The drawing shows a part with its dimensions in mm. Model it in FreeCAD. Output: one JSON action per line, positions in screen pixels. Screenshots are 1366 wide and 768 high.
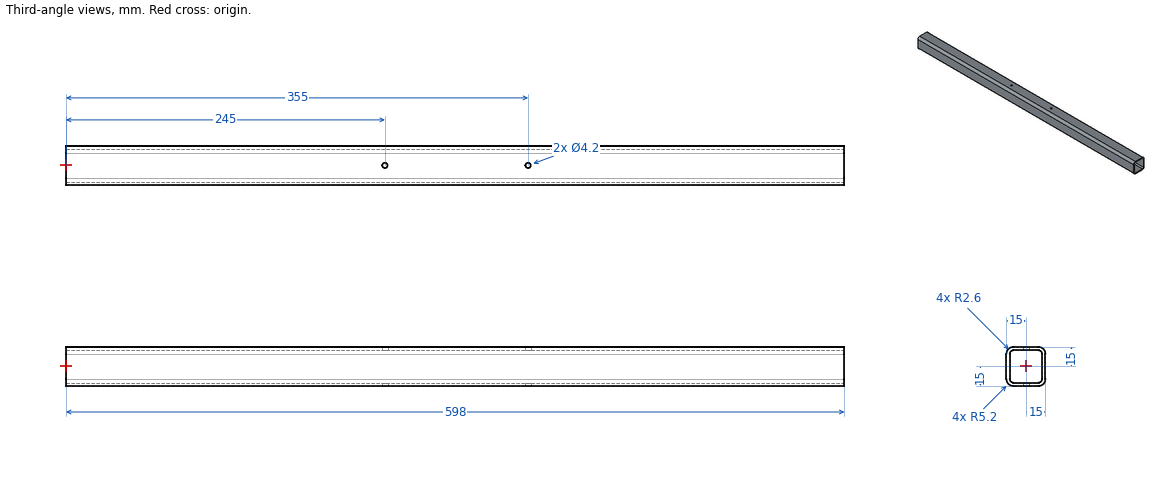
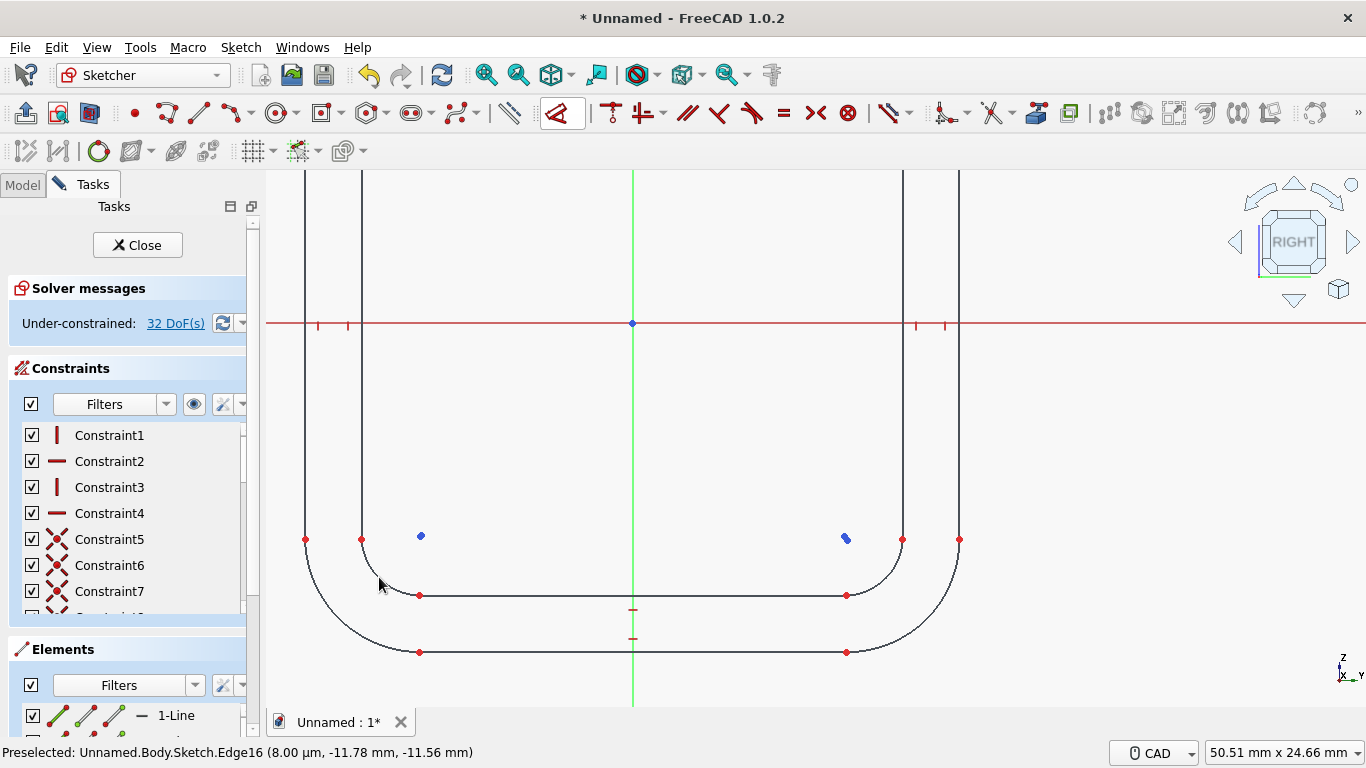
{"action": "left_click", "coordinate": [305, 239]}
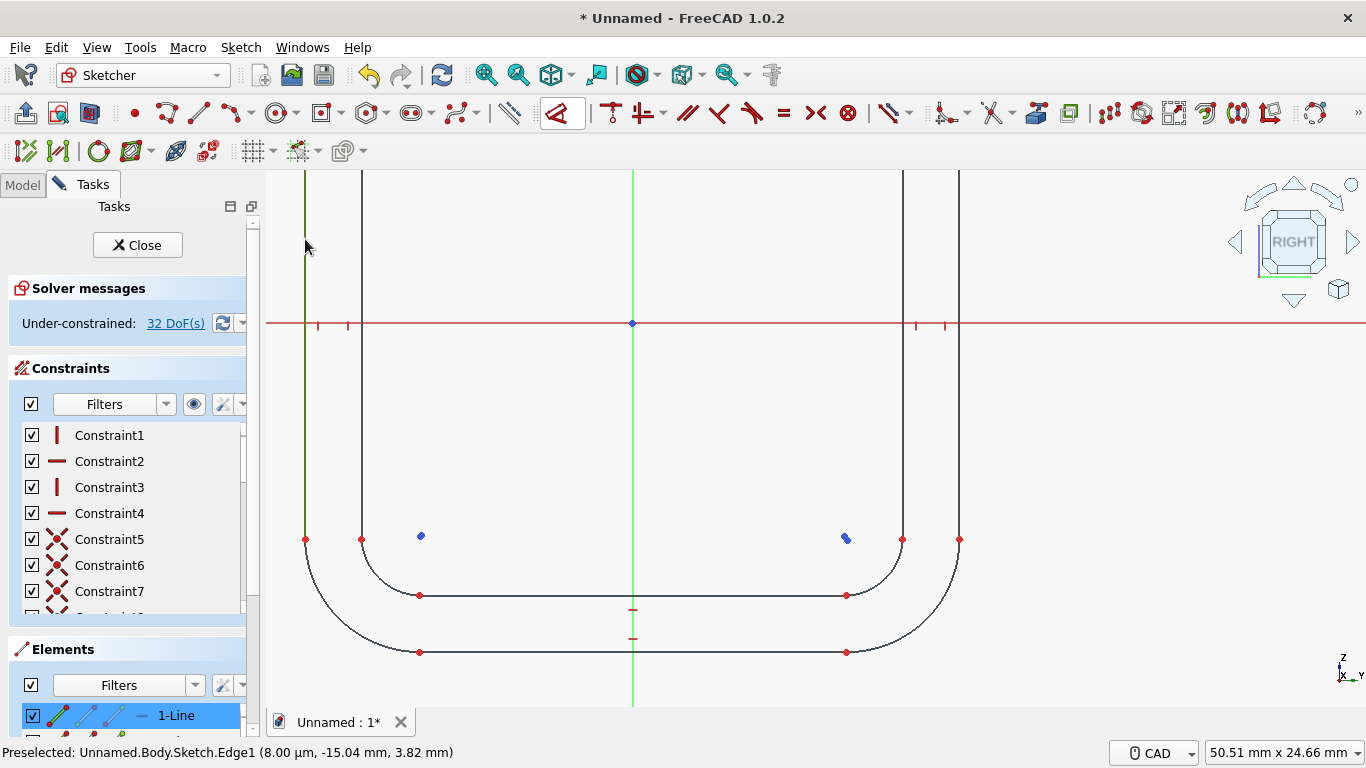
{"action": "left_click", "coordinate": [318, 590]}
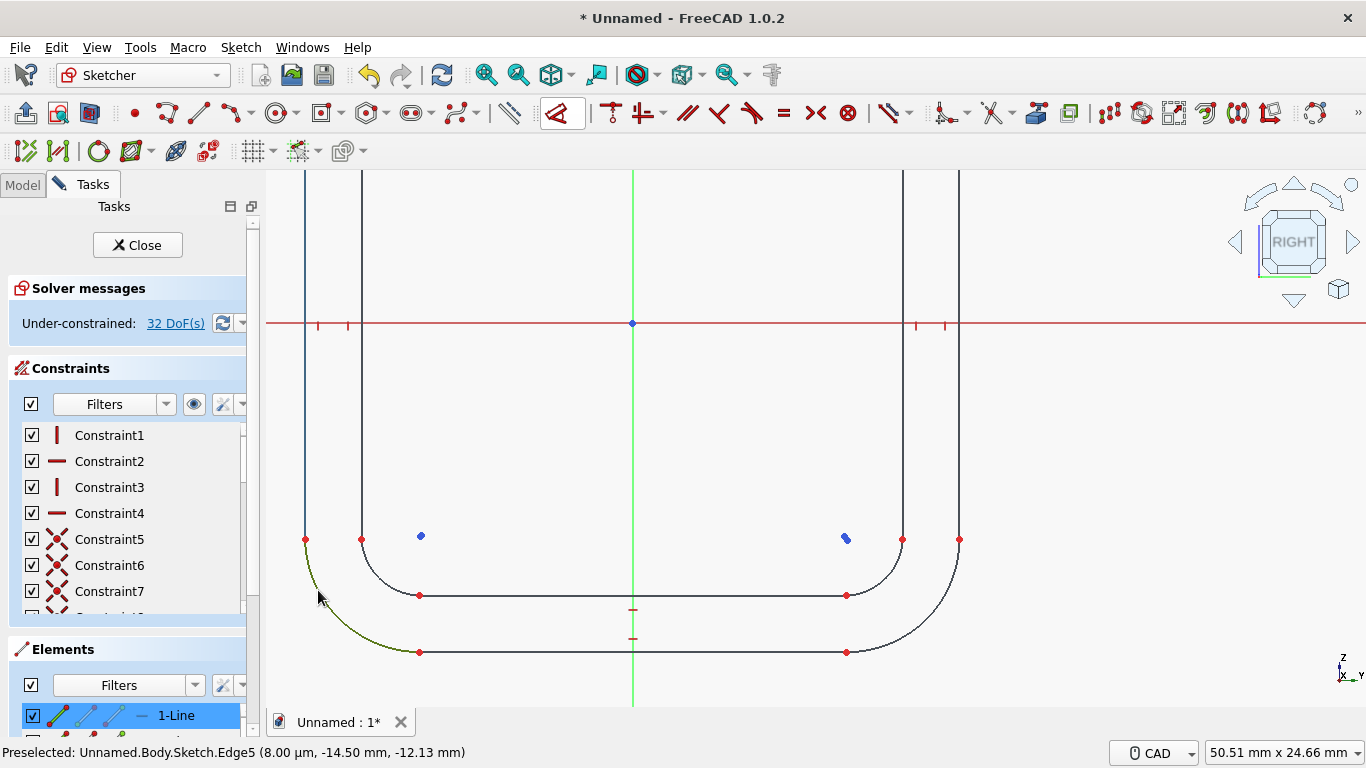
{"action": "key", "text": "t"}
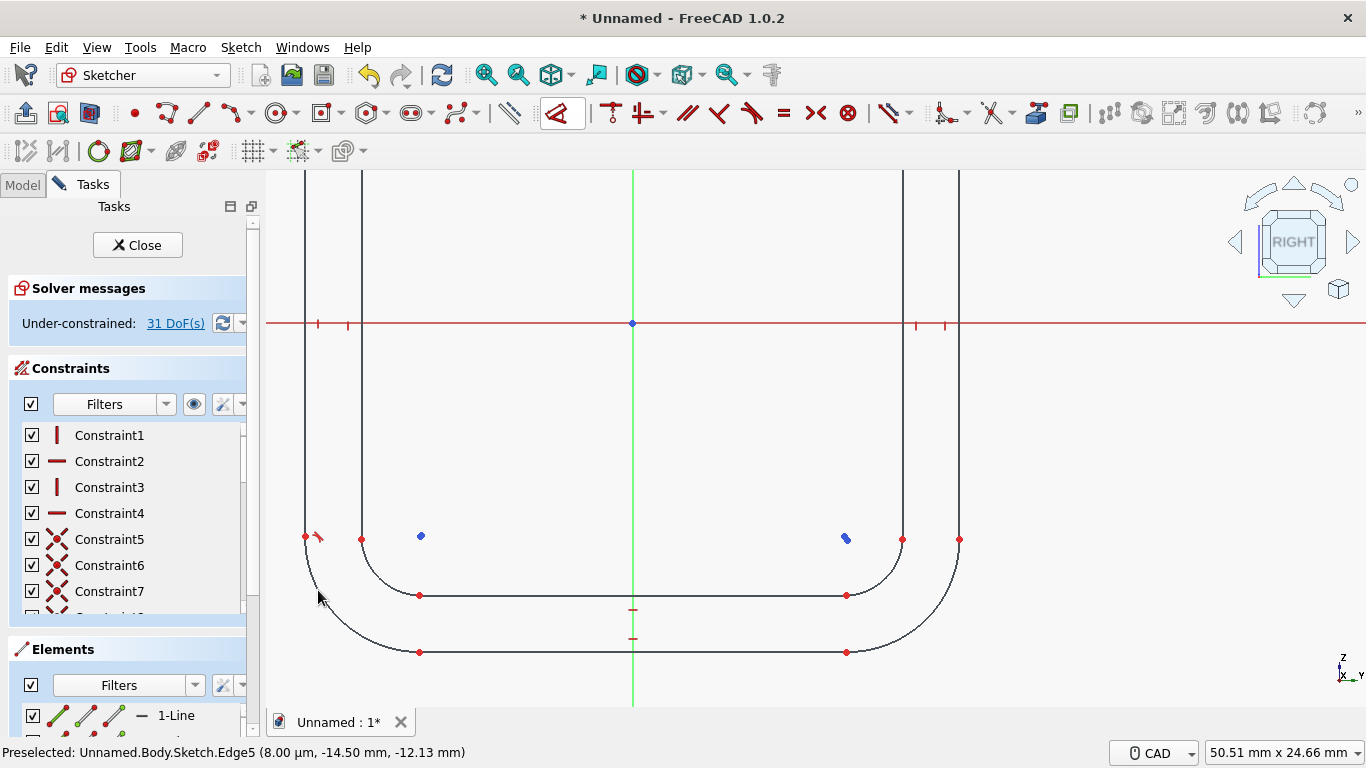
{"action": "left_click", "coordinate": [305, 239]}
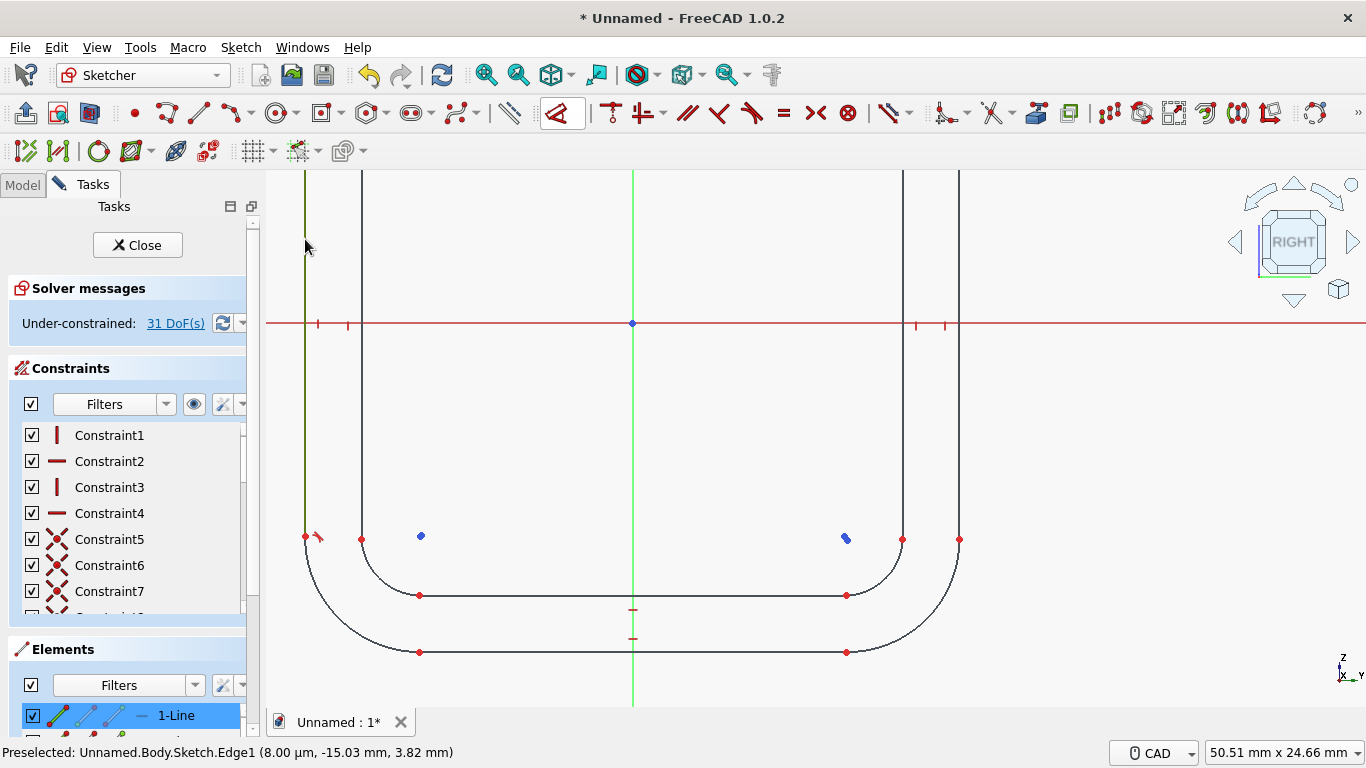
{"action": "scroll", "coordinate": [887, 579], "scroll_direction": "down", "scroll_amount": 3}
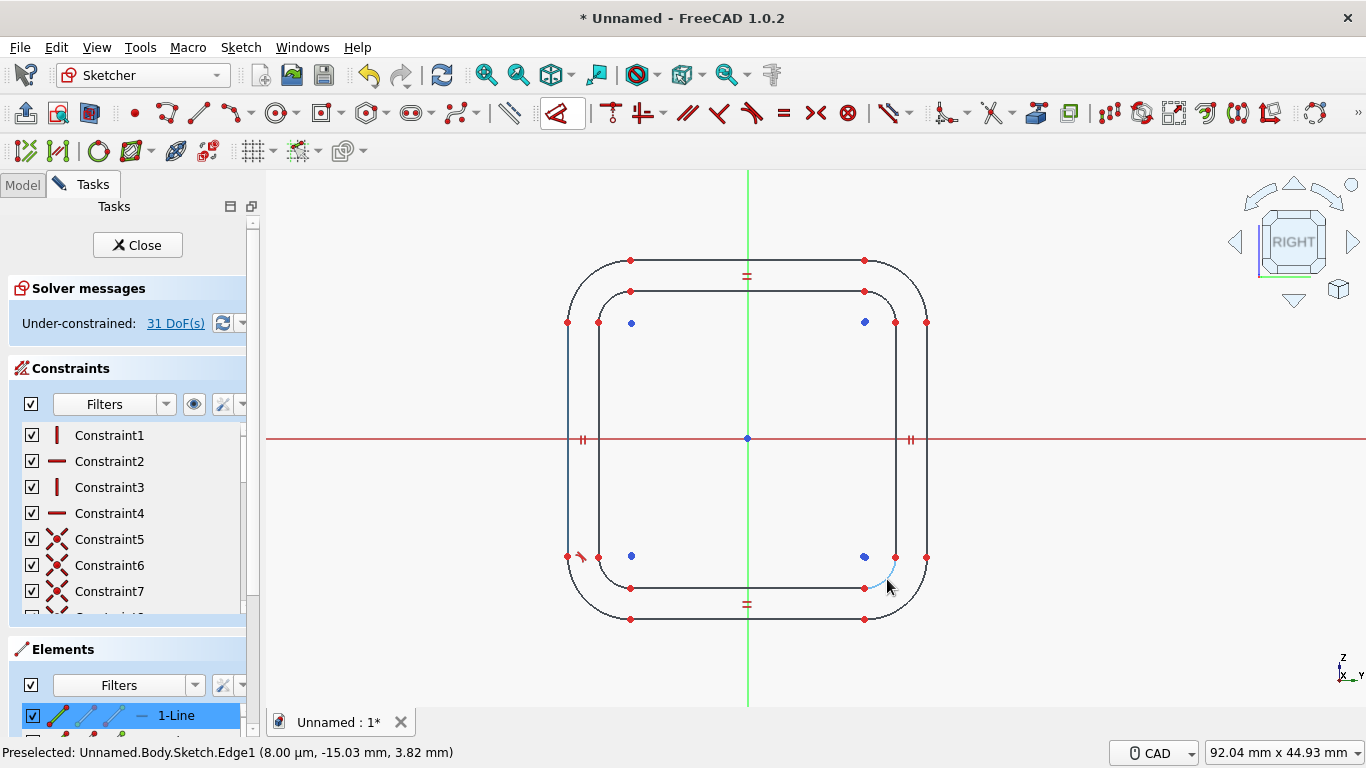
{"action": "left_click", "coordinate": [603, 267]}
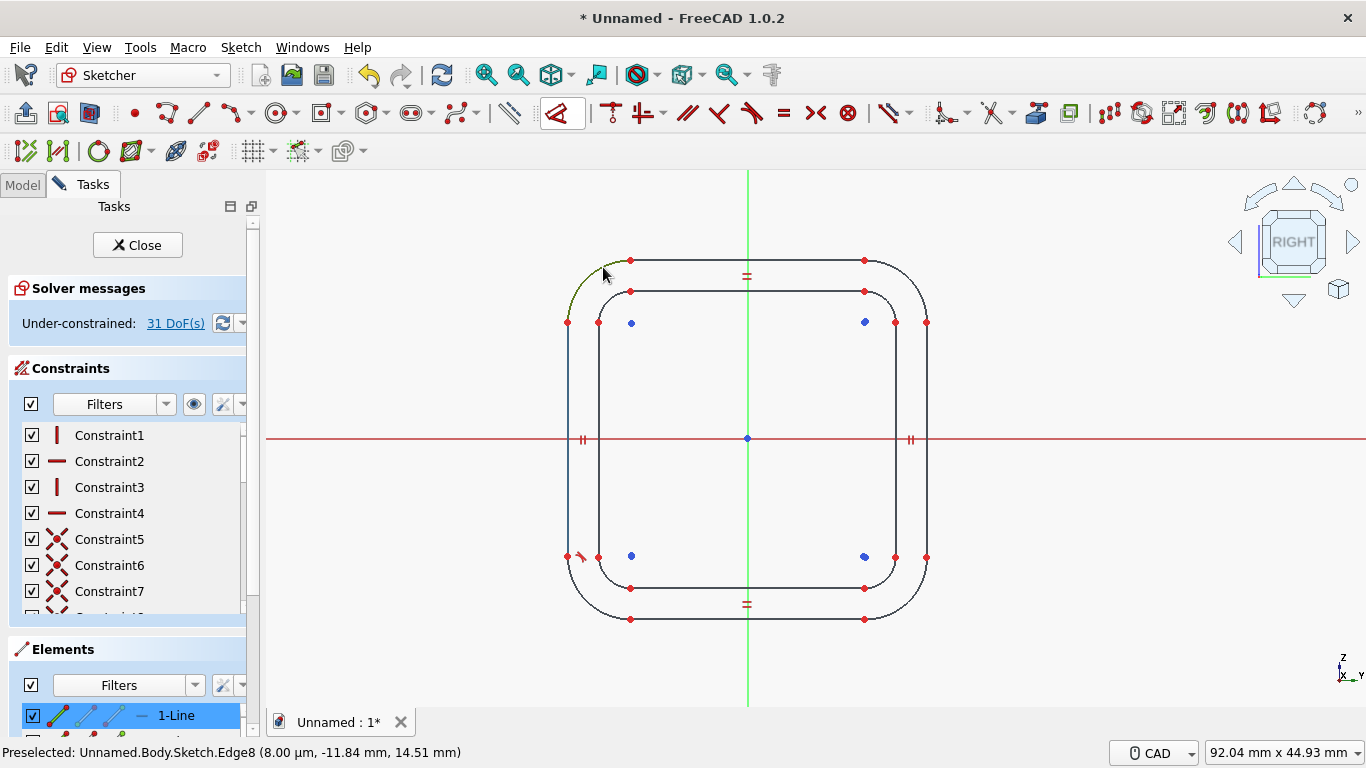
{"action": "left_click", "coordinate": [752, 114]}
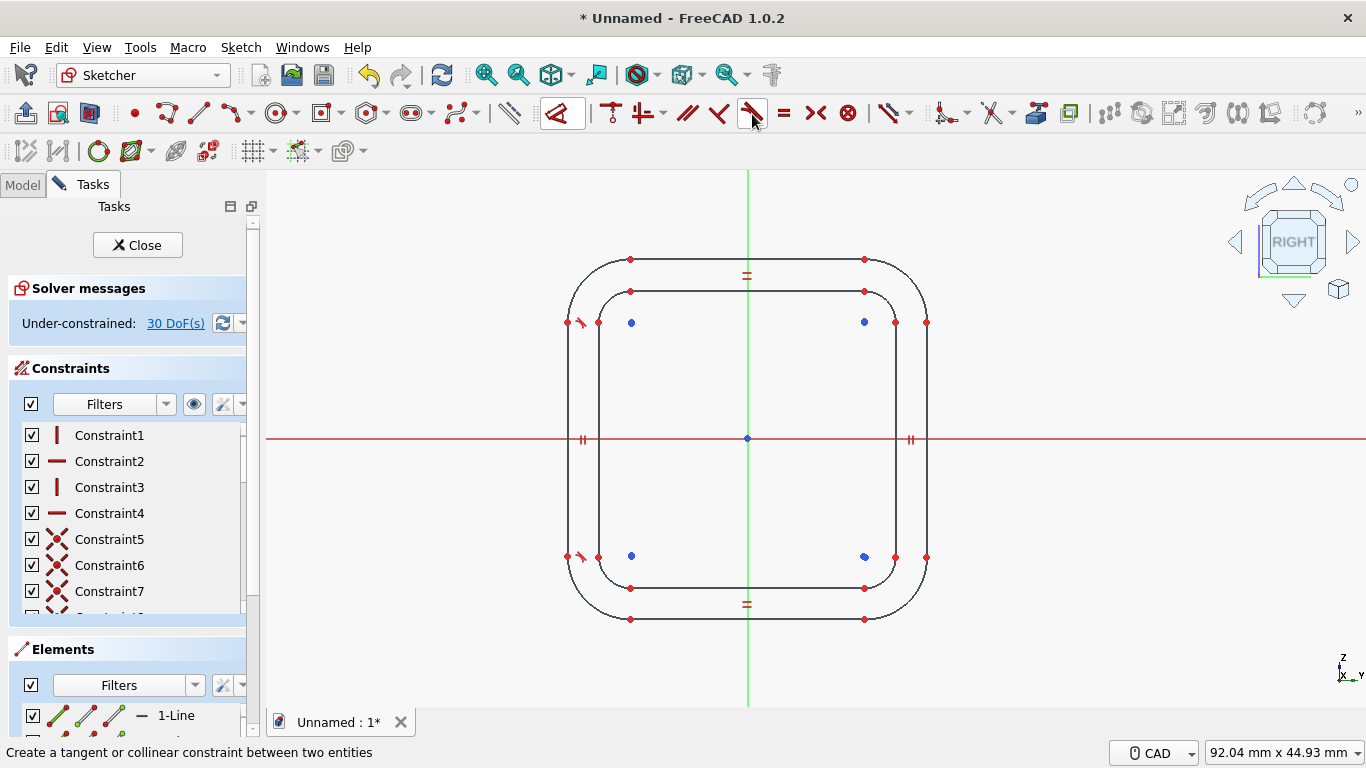
{"action": "left_click", "coordinate": [701, 619]}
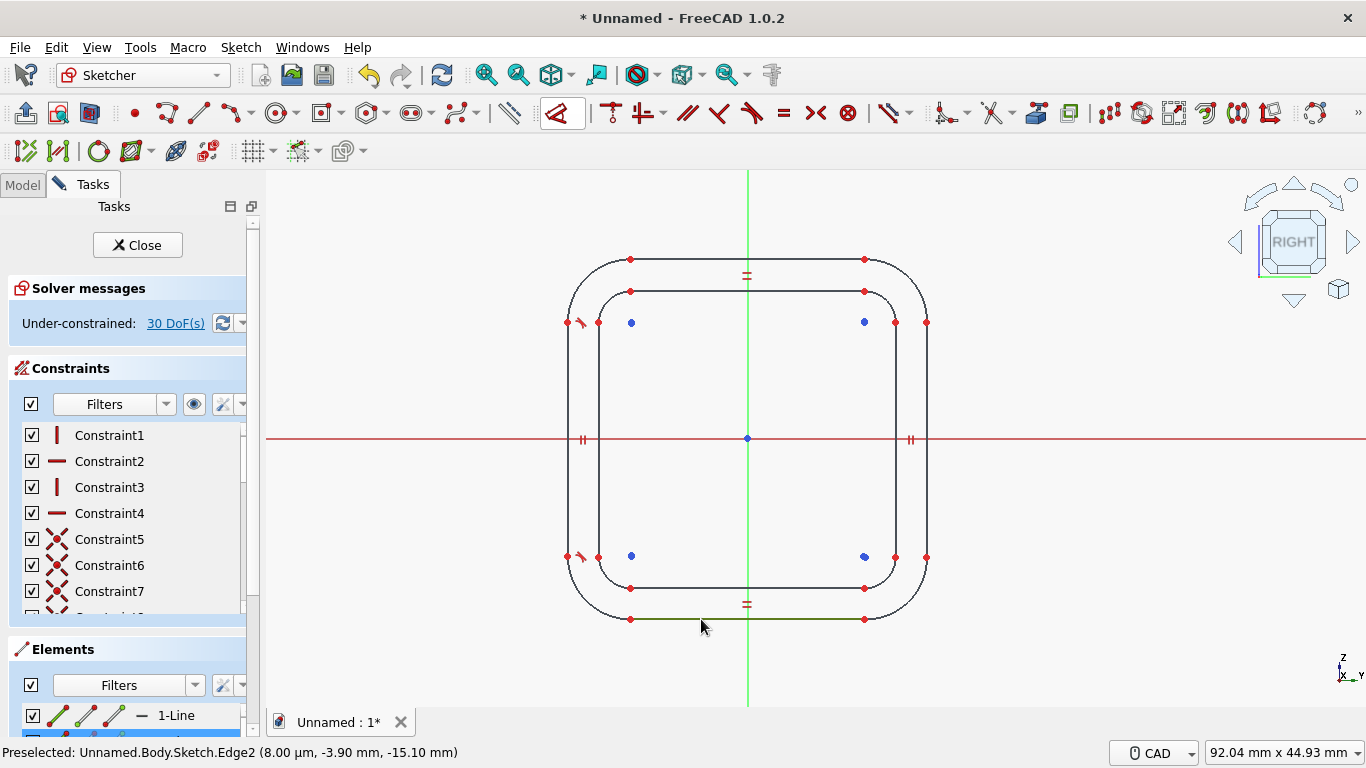
{"action": "left_click", "coordinate": [575, 585]}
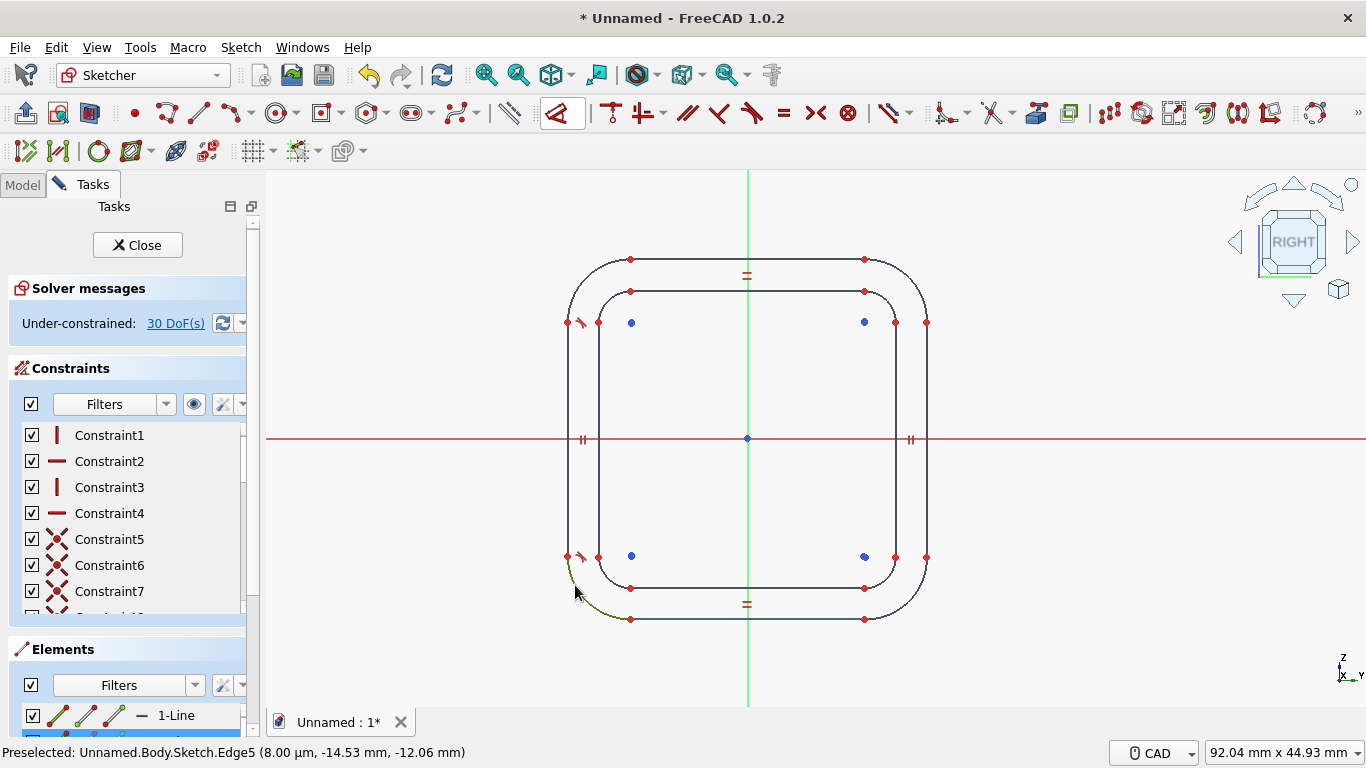
{"action": "left_click", "coordinate": [752, 114]}